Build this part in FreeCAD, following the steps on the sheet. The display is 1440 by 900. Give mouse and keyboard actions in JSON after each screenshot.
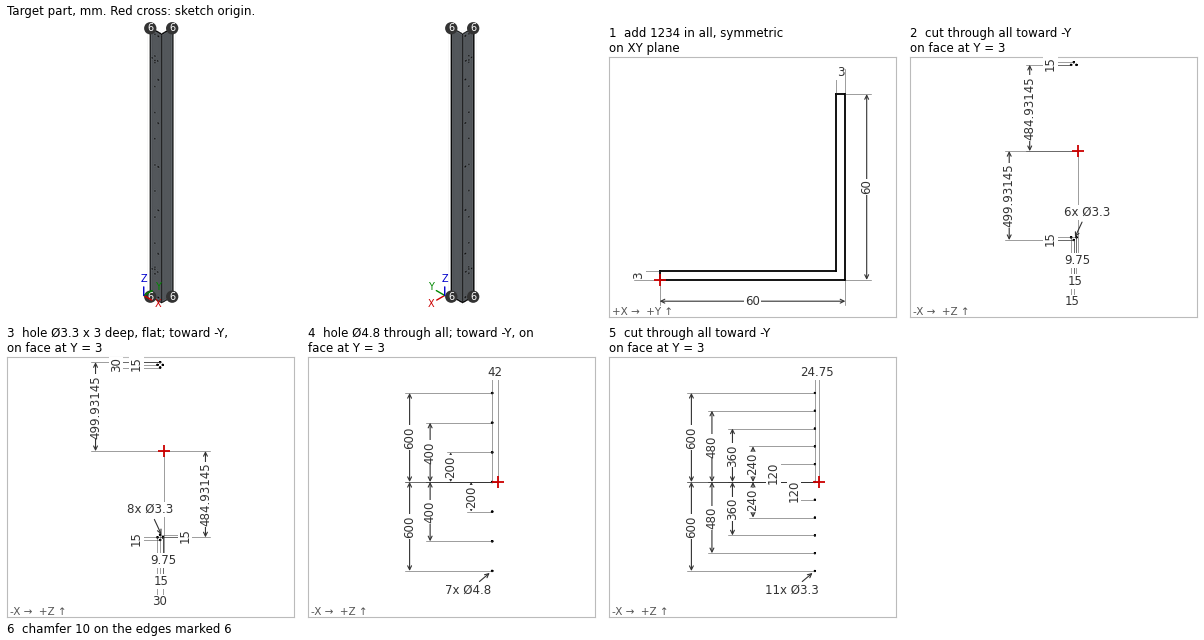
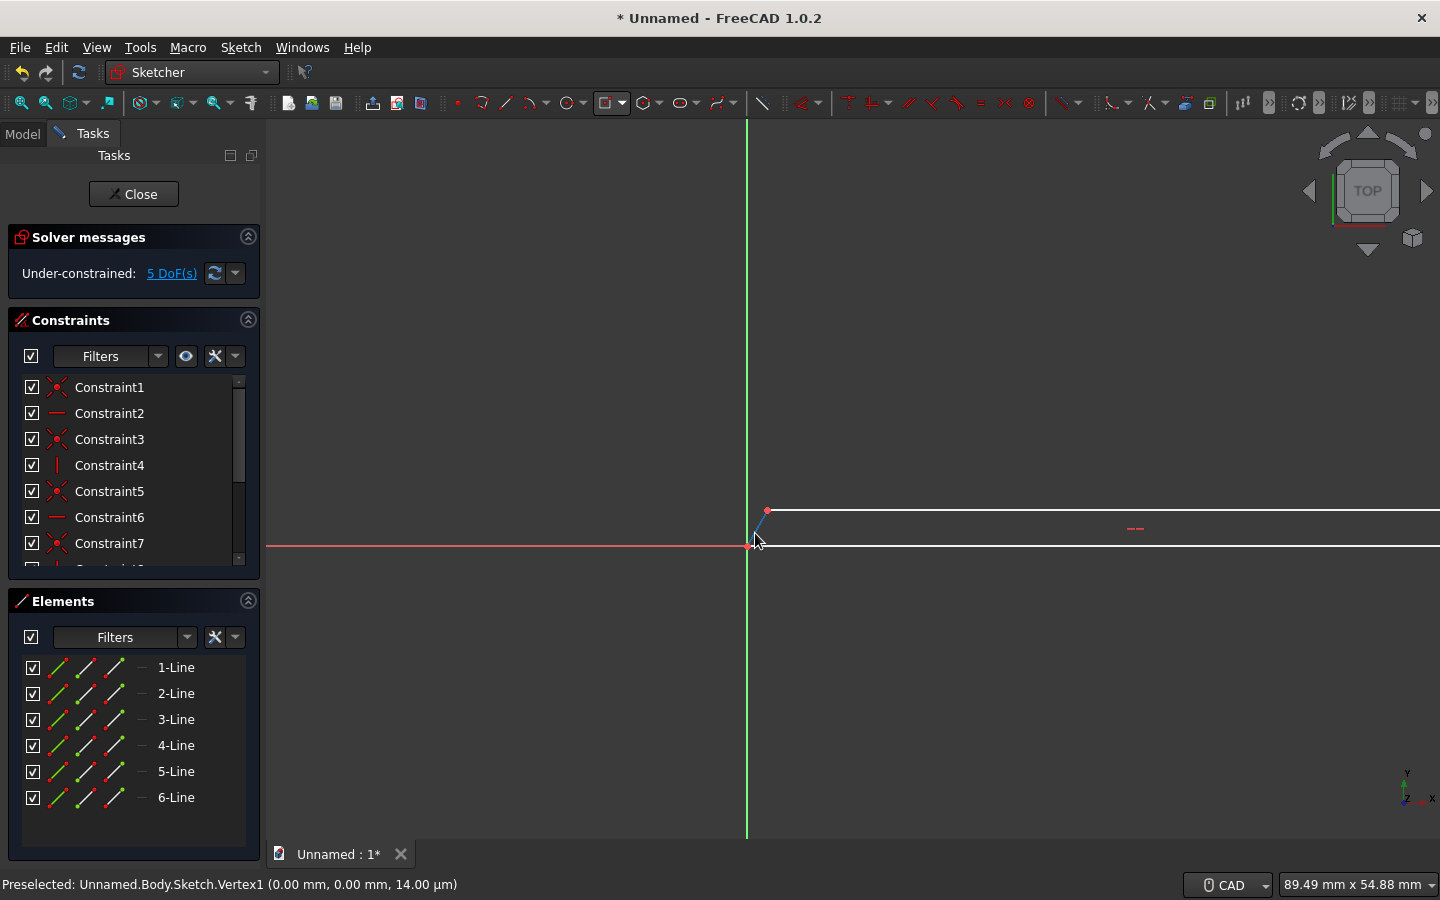
{"action": "left_click", "coordinate": [755, 532]}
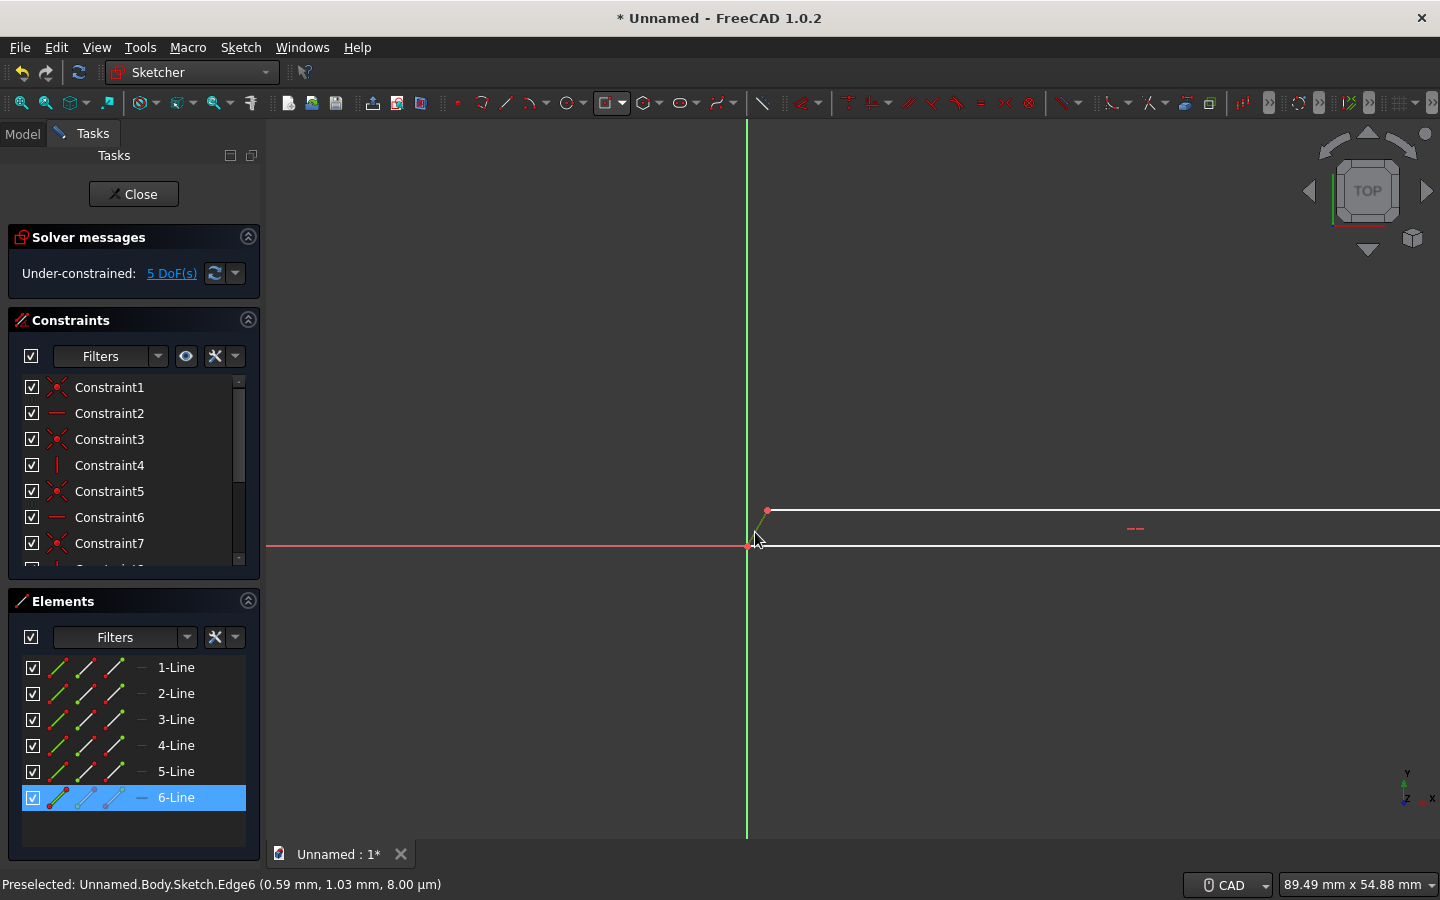
{"action": "key", "text": "v"}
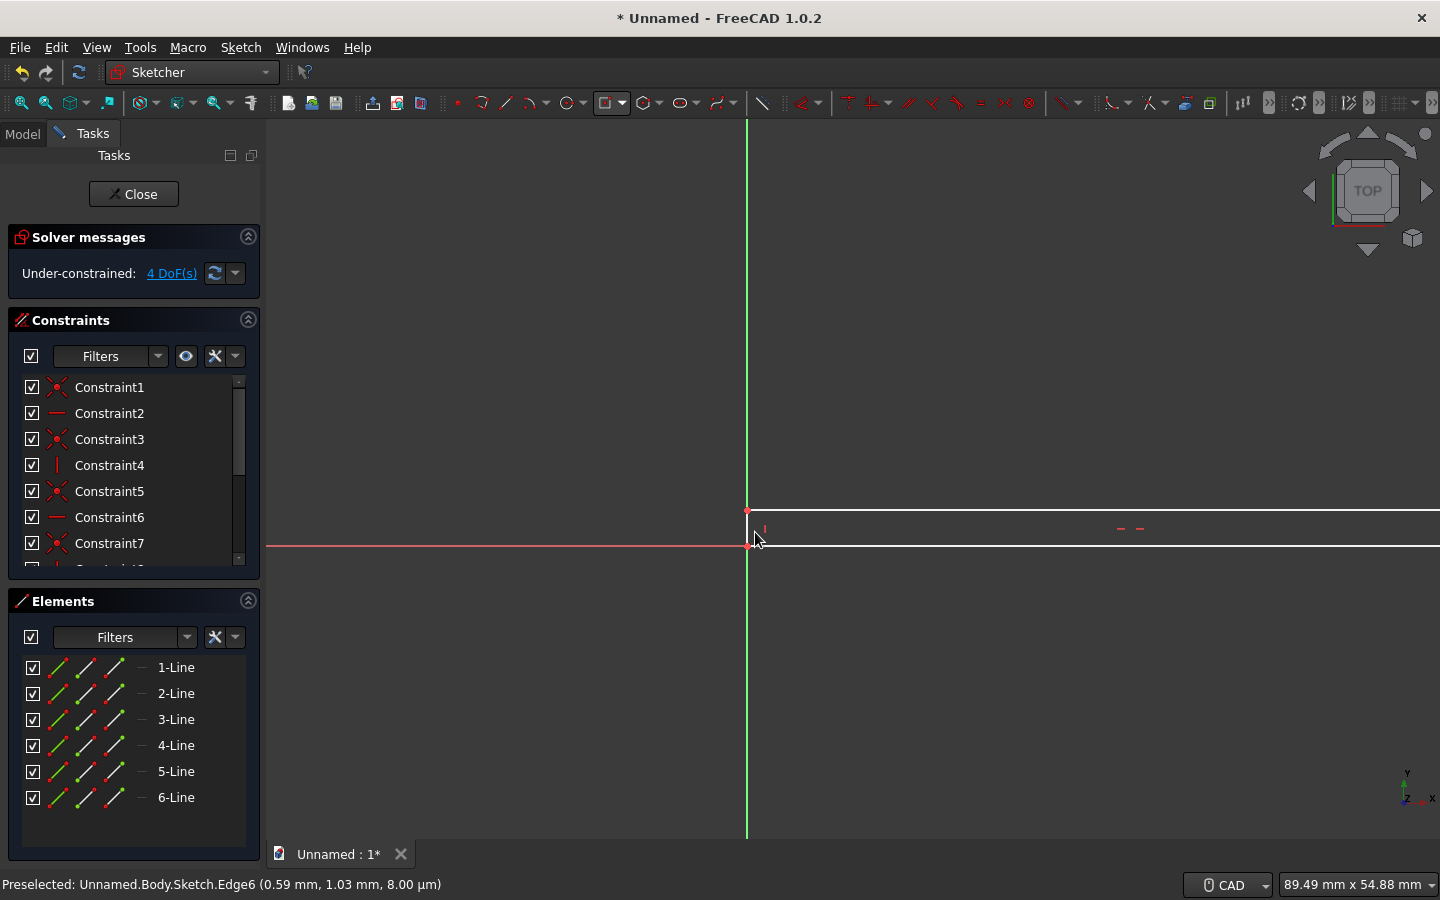
{"action": "left_click", "coordinate": [802, 104]}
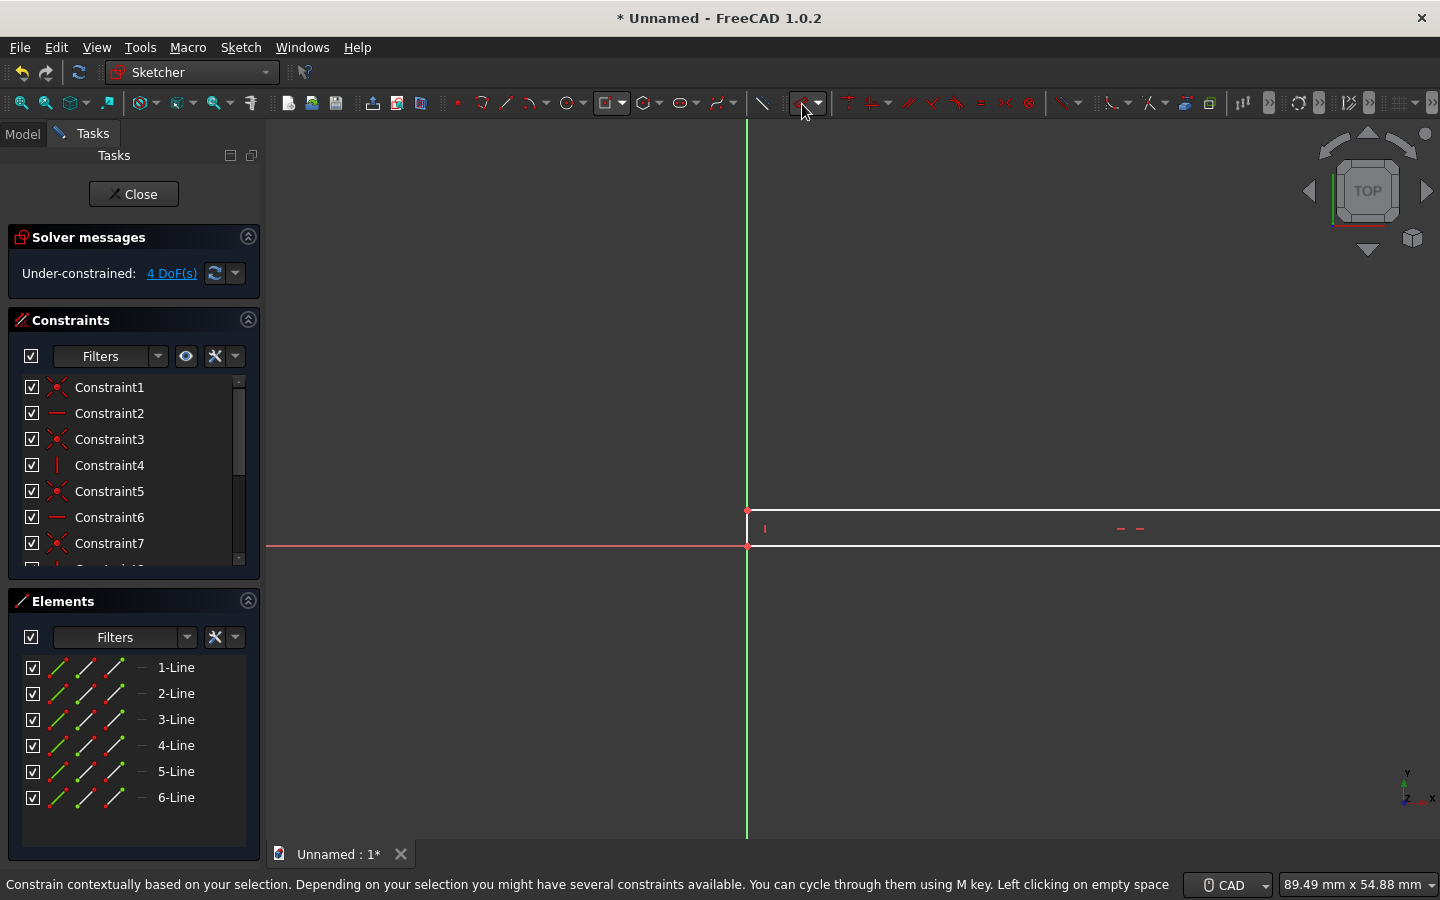
{"action": "scroll", "coordinate": [351, 811], "scroll_direction": "down", "scroll_amount": 3}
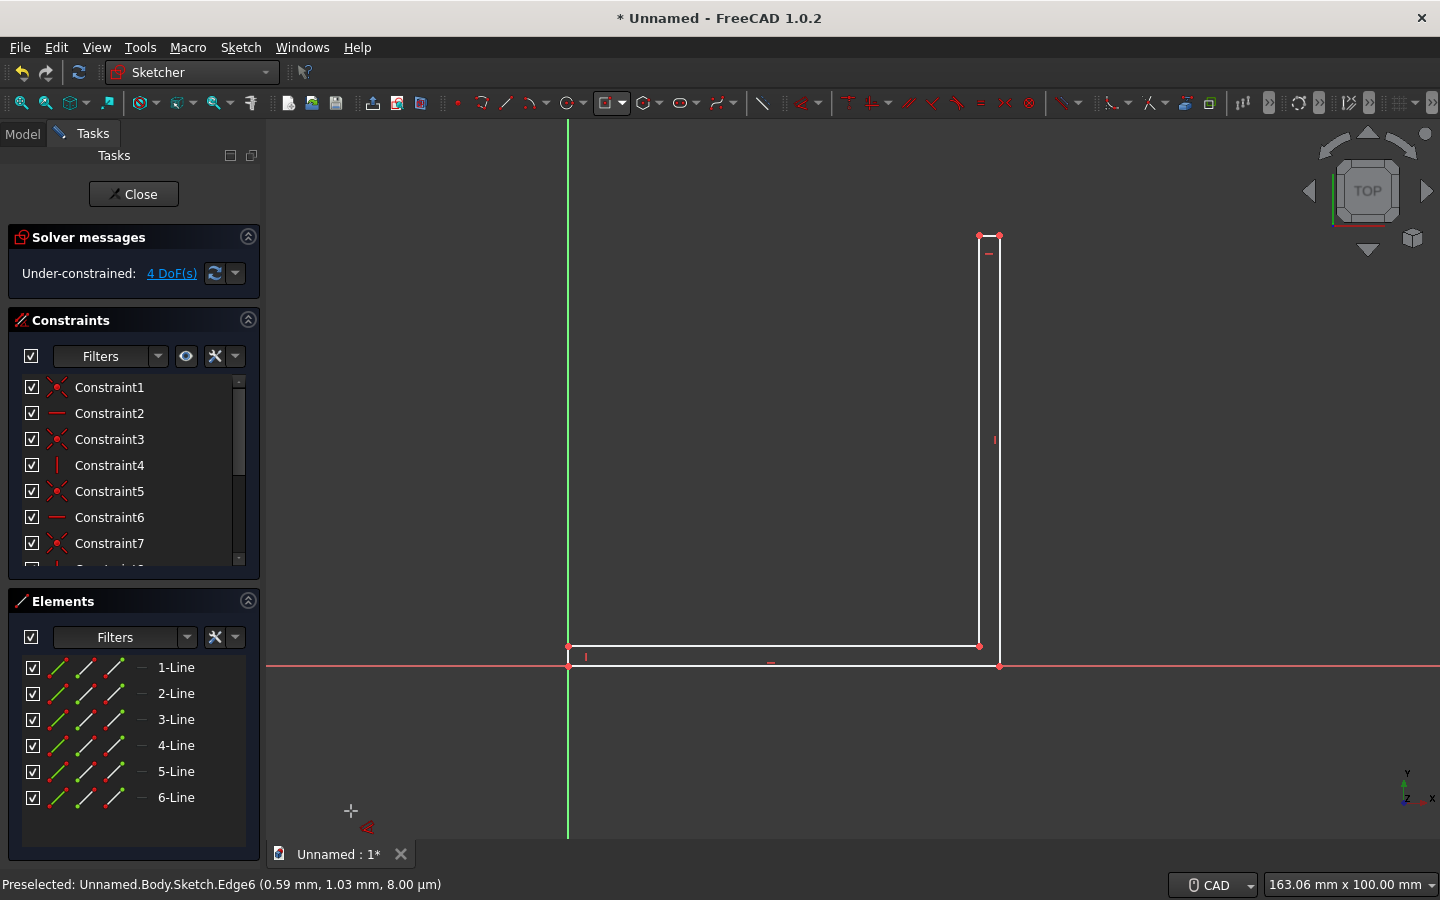
{"action": "scroll", "coordinate": [994, 236], "scroll_direction": "up", "scroll_amount": 4}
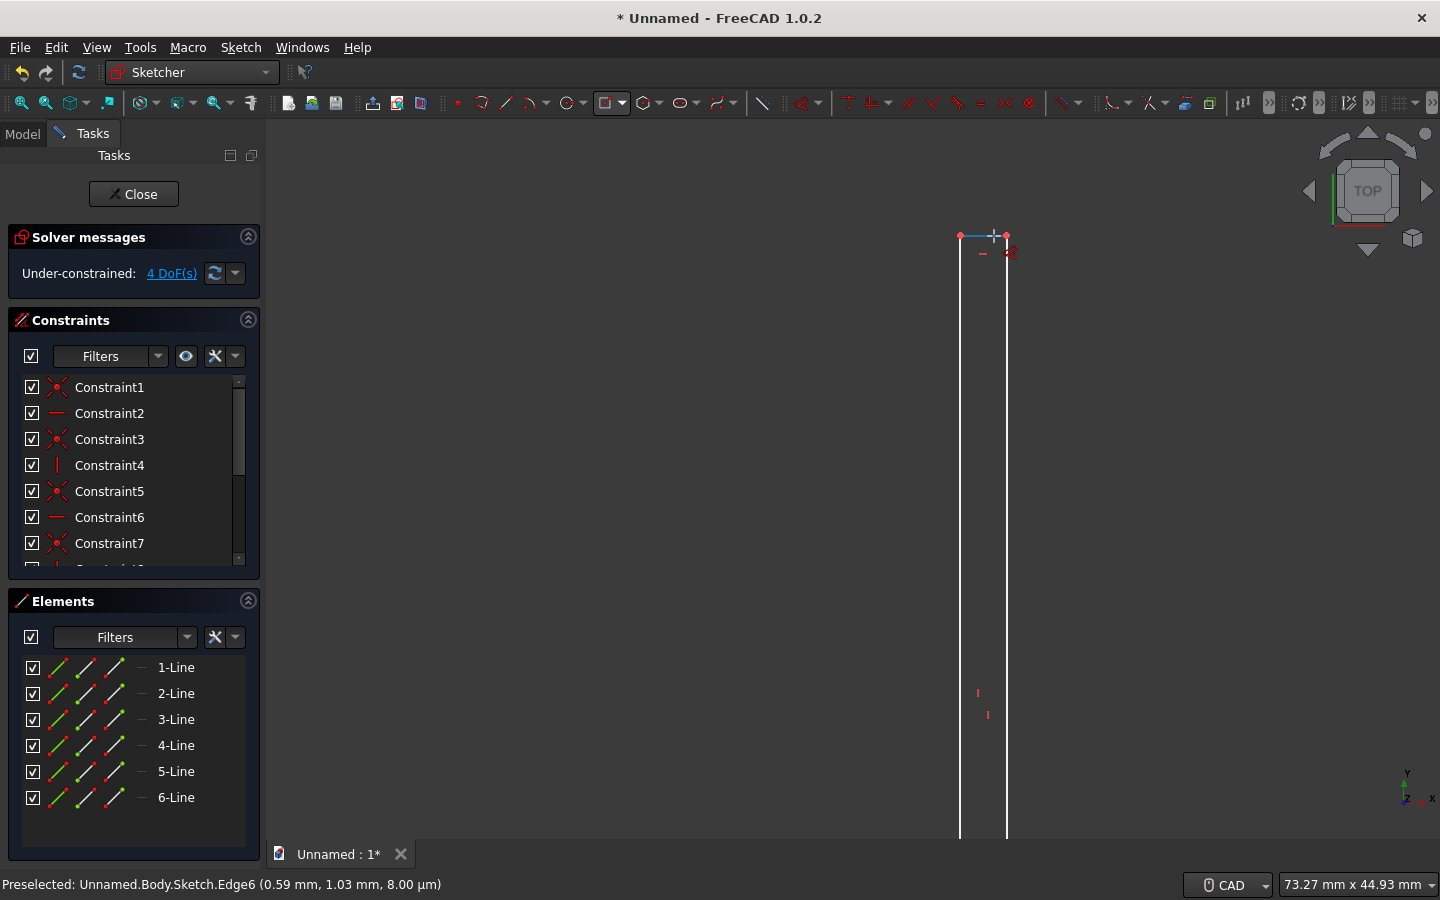
{"action": "left_click", "coordinate": [993, 236]}
{"action": "left_click", "coordinate": [983, 202]}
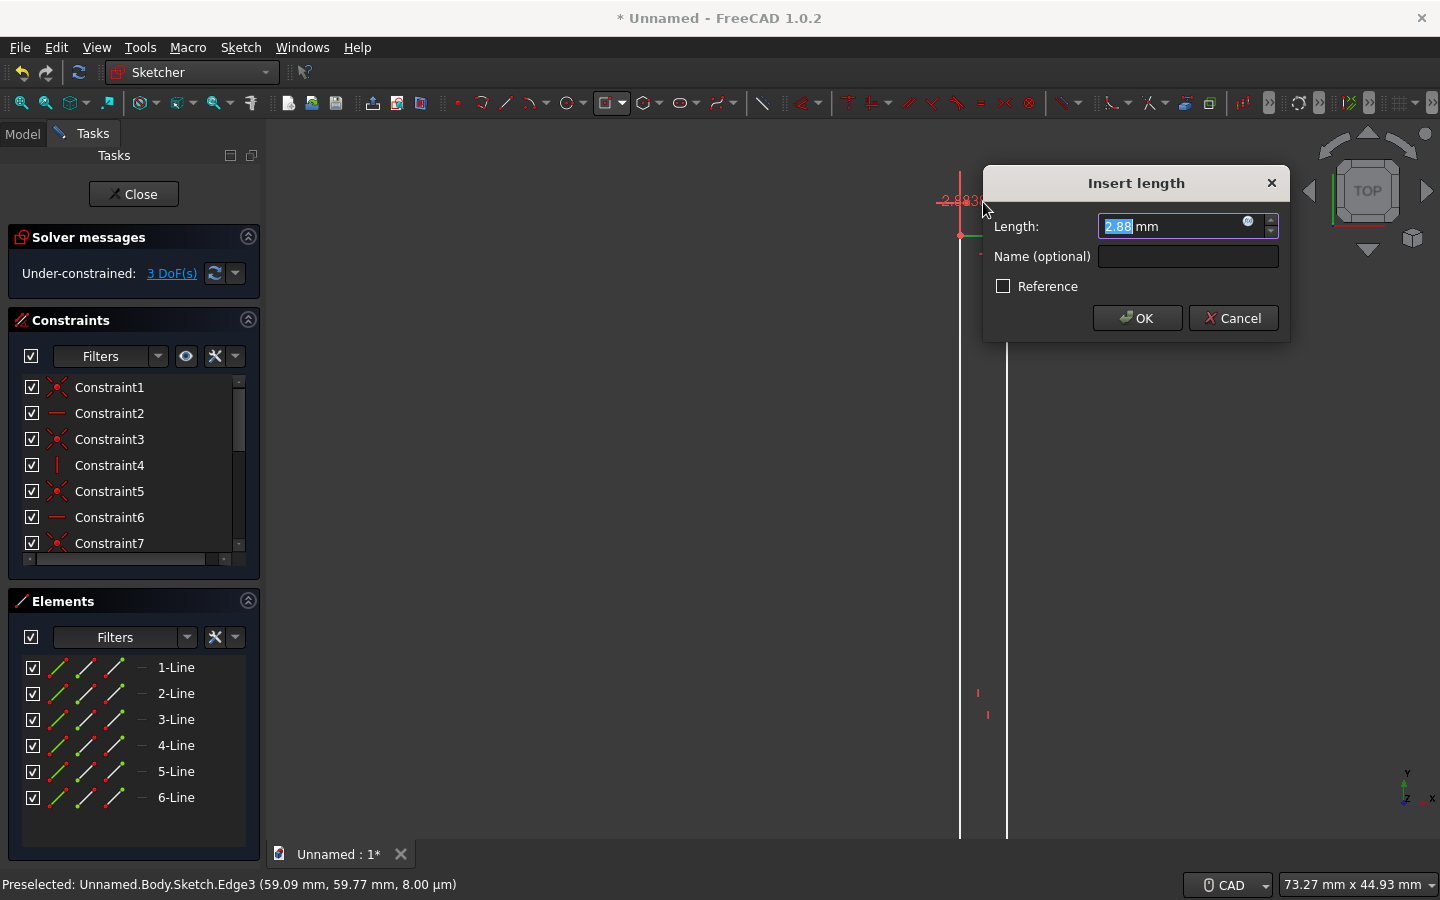
{"action": "type", "text": "3"}
{"action": "key", "text": "Return"}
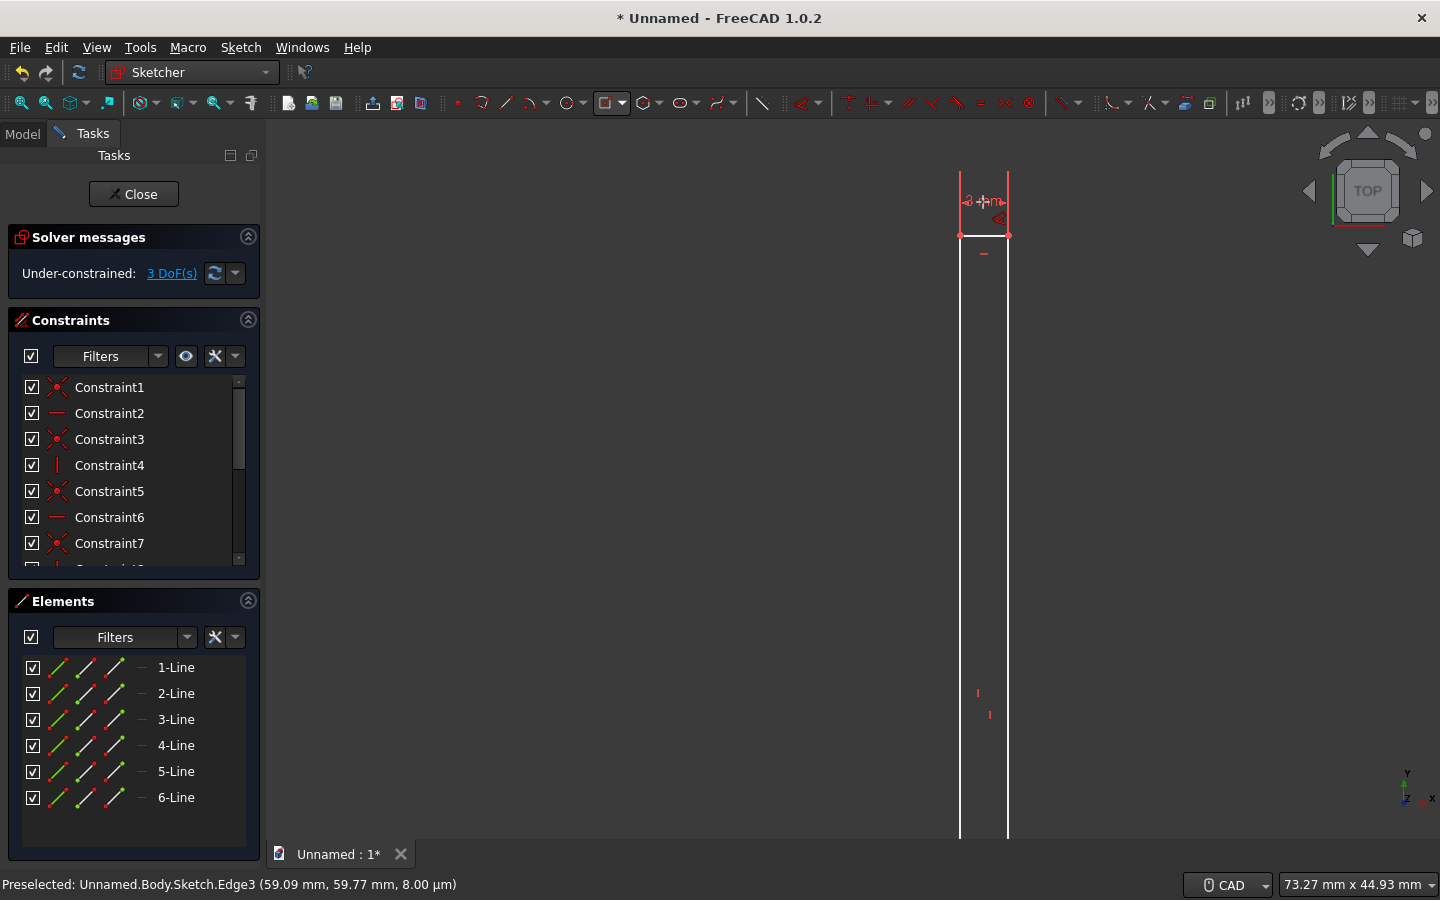
{"action": "scroll", "coordinate": [995, 288], "scroll_direction": "down", "scroll_amount": 4}